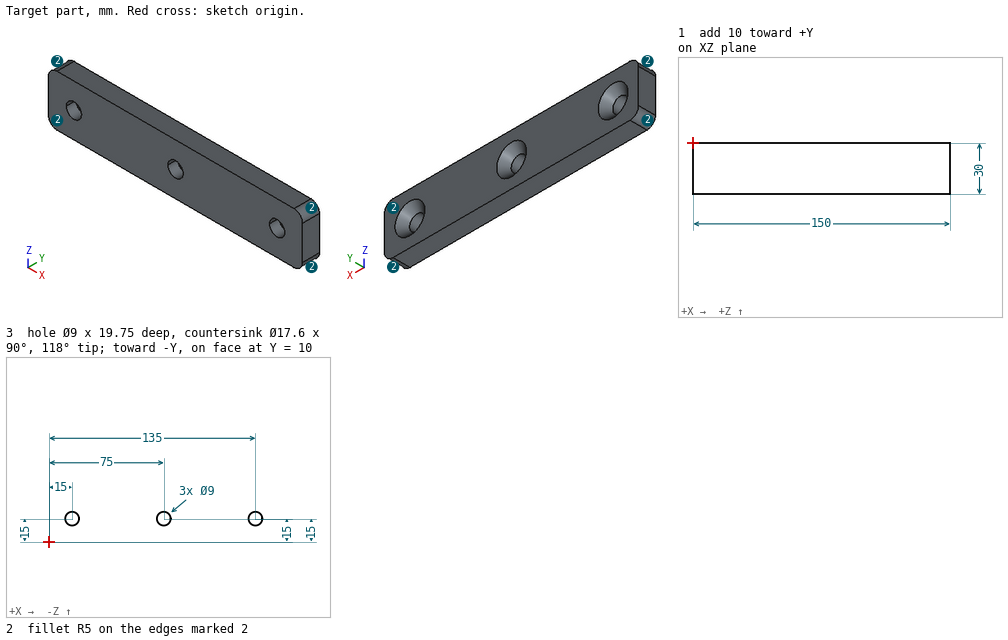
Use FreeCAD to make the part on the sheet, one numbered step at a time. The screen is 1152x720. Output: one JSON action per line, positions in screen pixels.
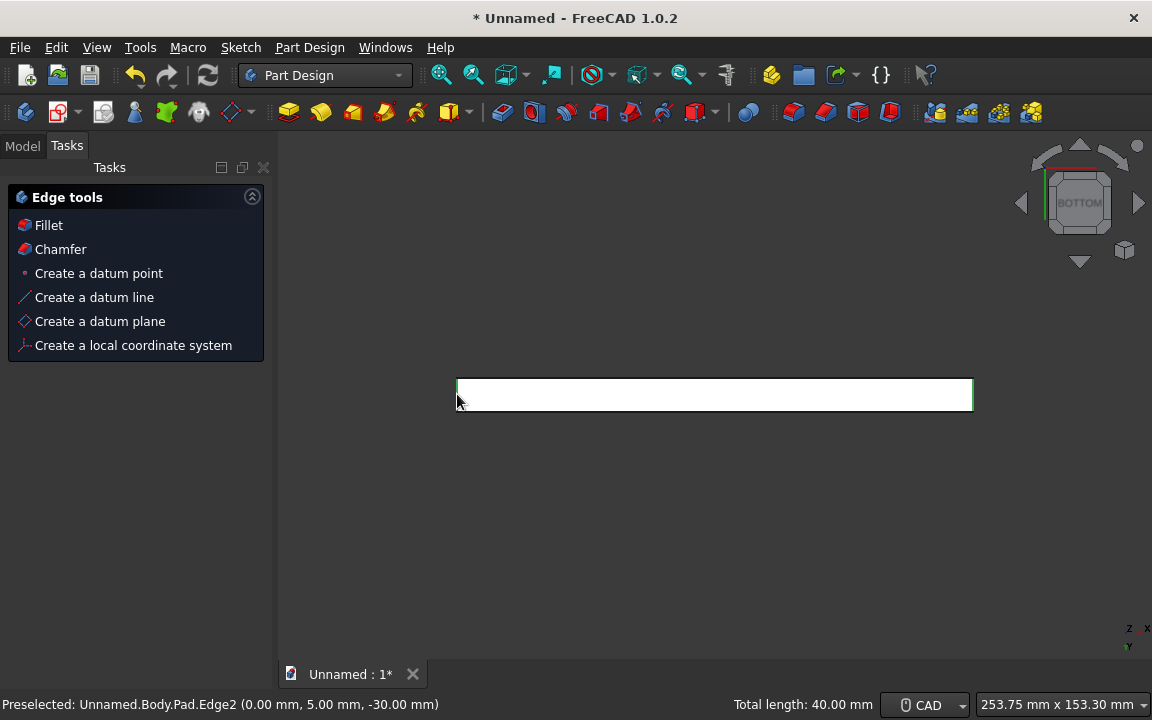
{"action": "left_click", "coordinate": [794, 112]}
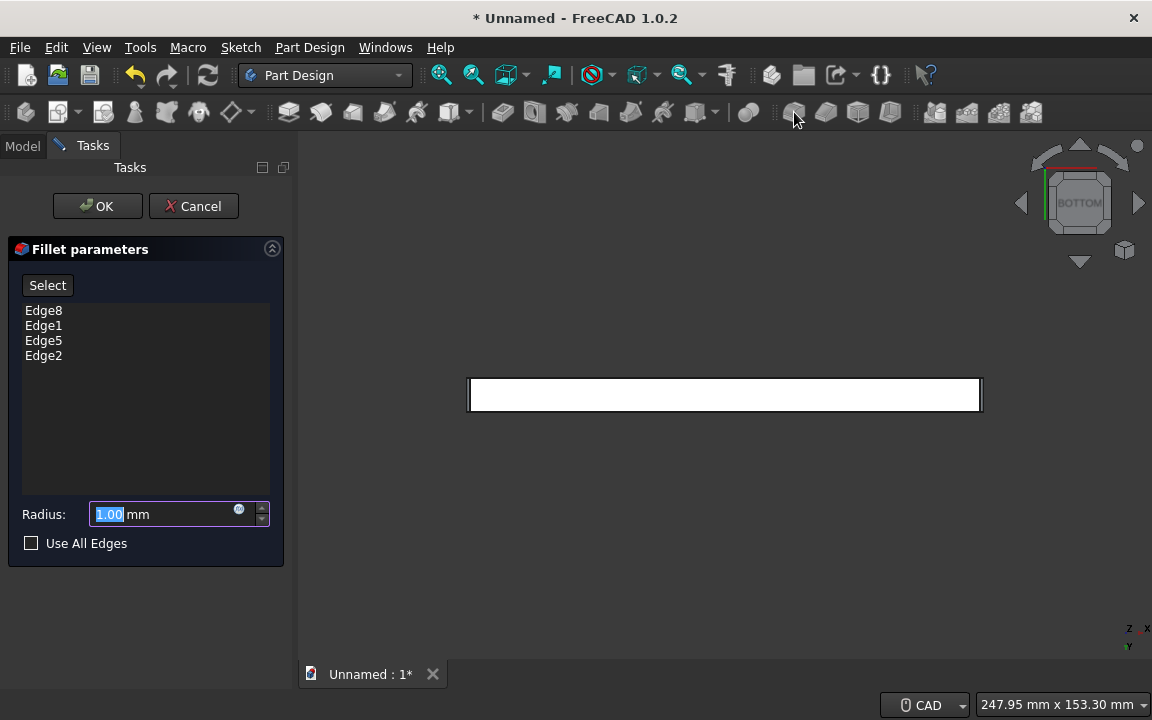
{"action": "type", "text": "5"}
{"action": "key", "text": "Tab"}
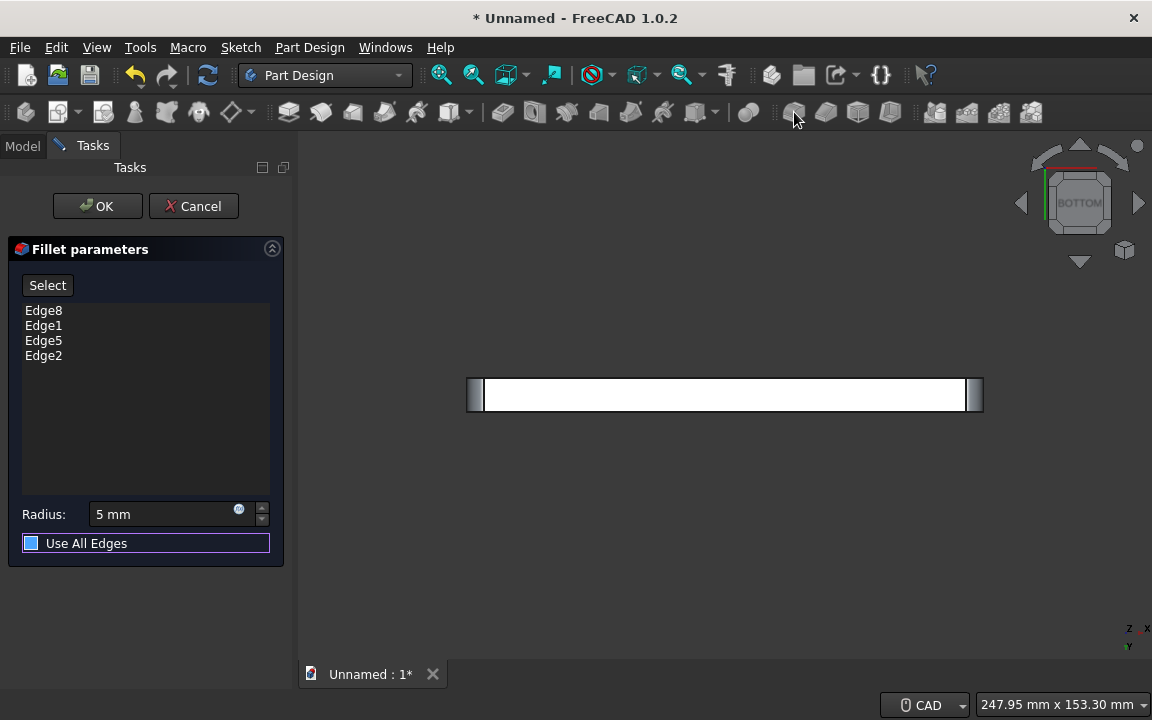
{"action": "left_click", "coordinate": [98, 206]}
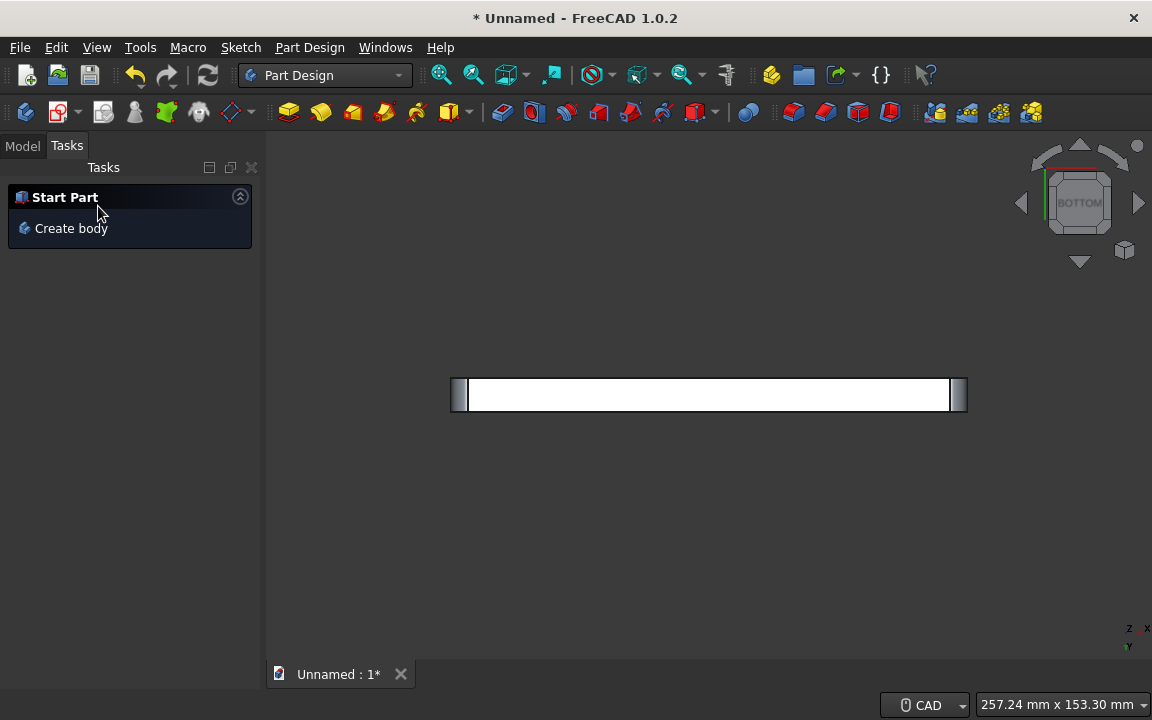
{"action": "key", "text": "4"}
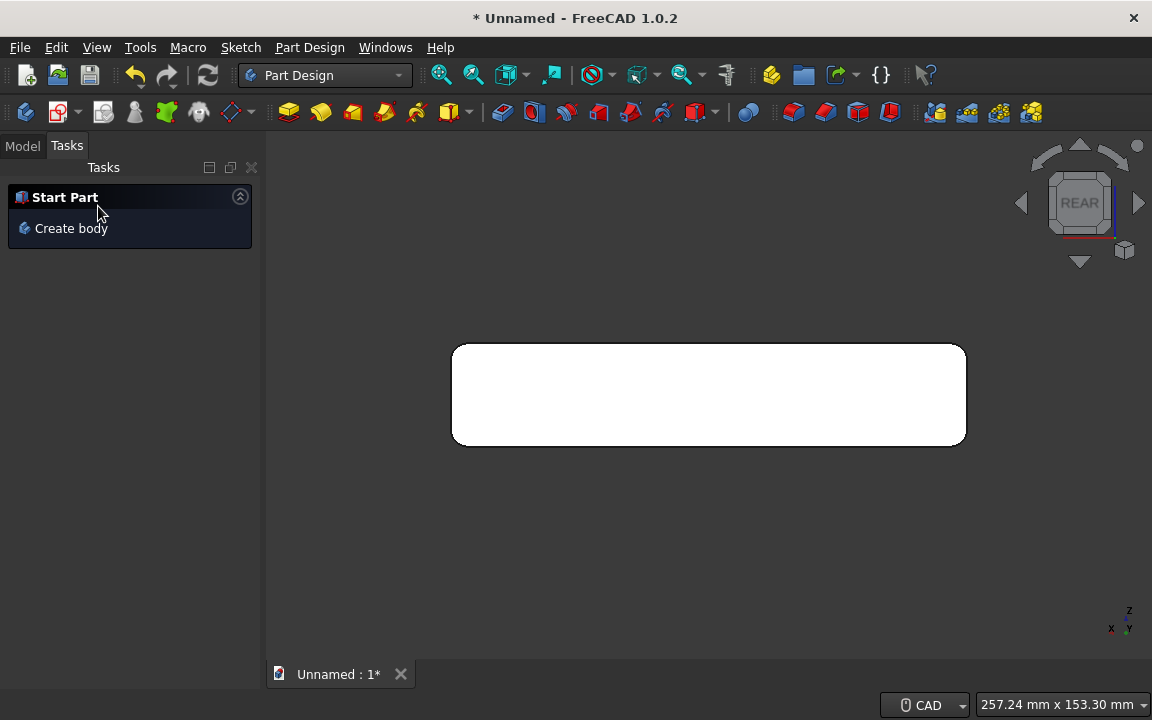
{"action": "left_click", "coordinate": [561, 394]}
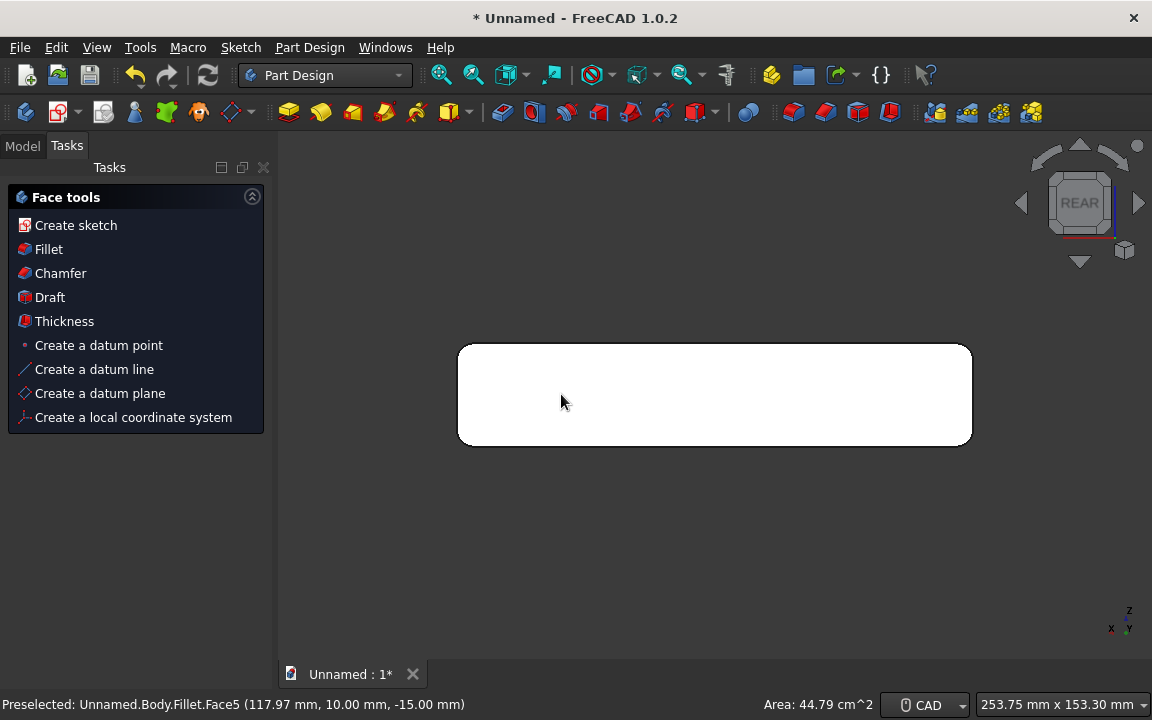
{"action": "left_click", "coordinate": [58, 112]}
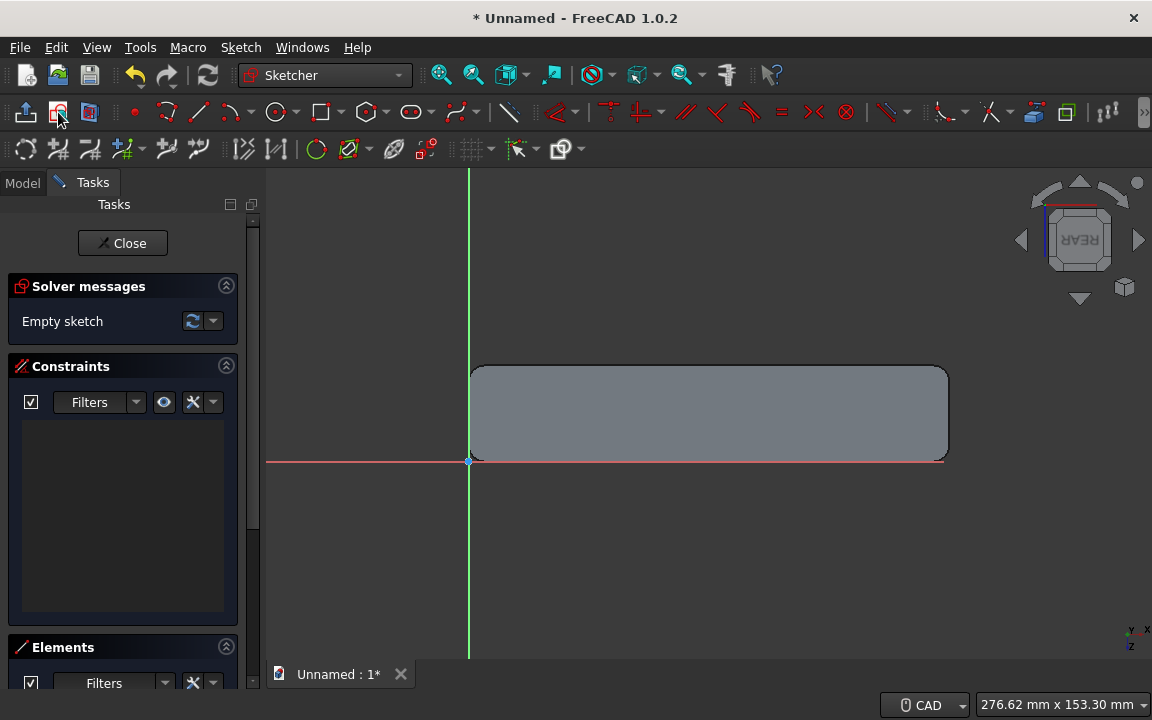
{"action": "left_click", "coordinate": [276, 112]}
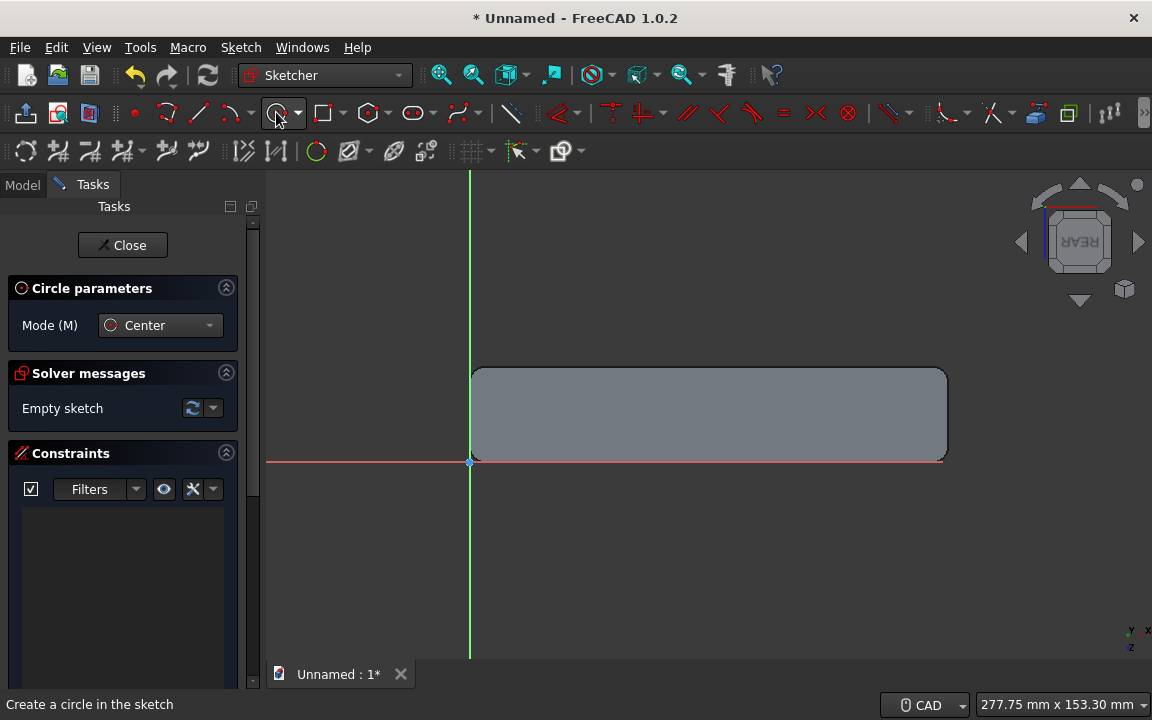
{"action": "scroll", "coordinate": [709, 415], "scroll_direction": "up", "scroll_amount": 3}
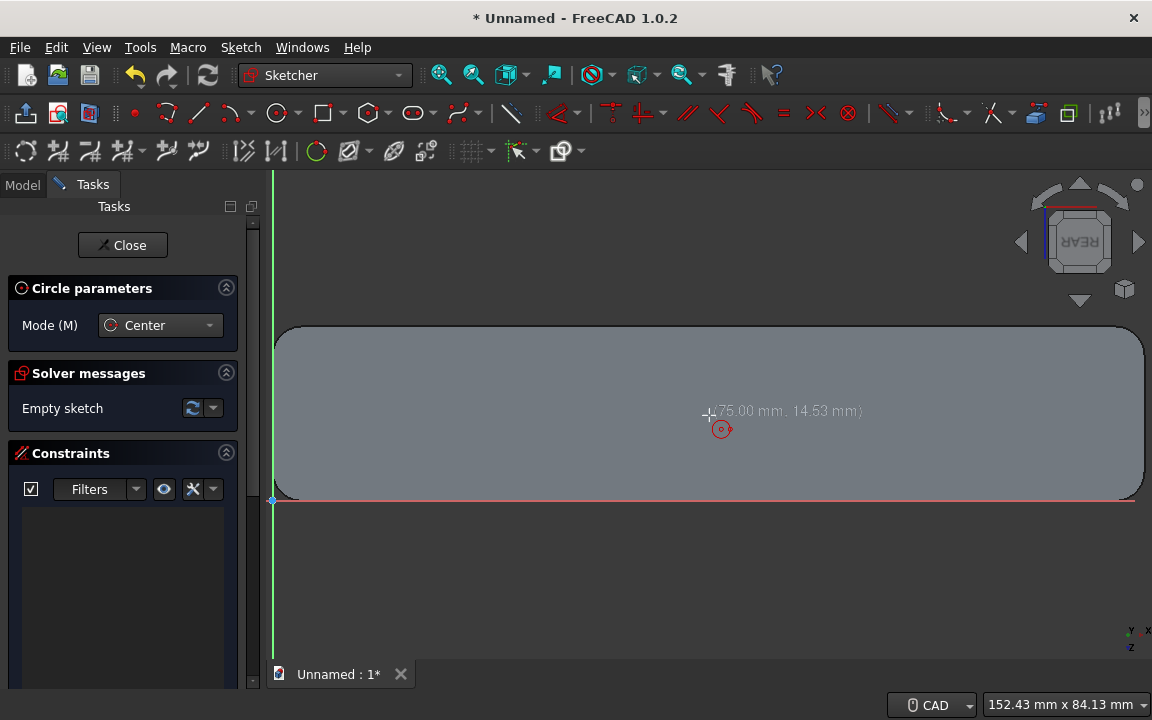
{"action": "left_click", "coordinate": [709, 414]}
{"action": "mouse_move", "coordinate": [727, 395]}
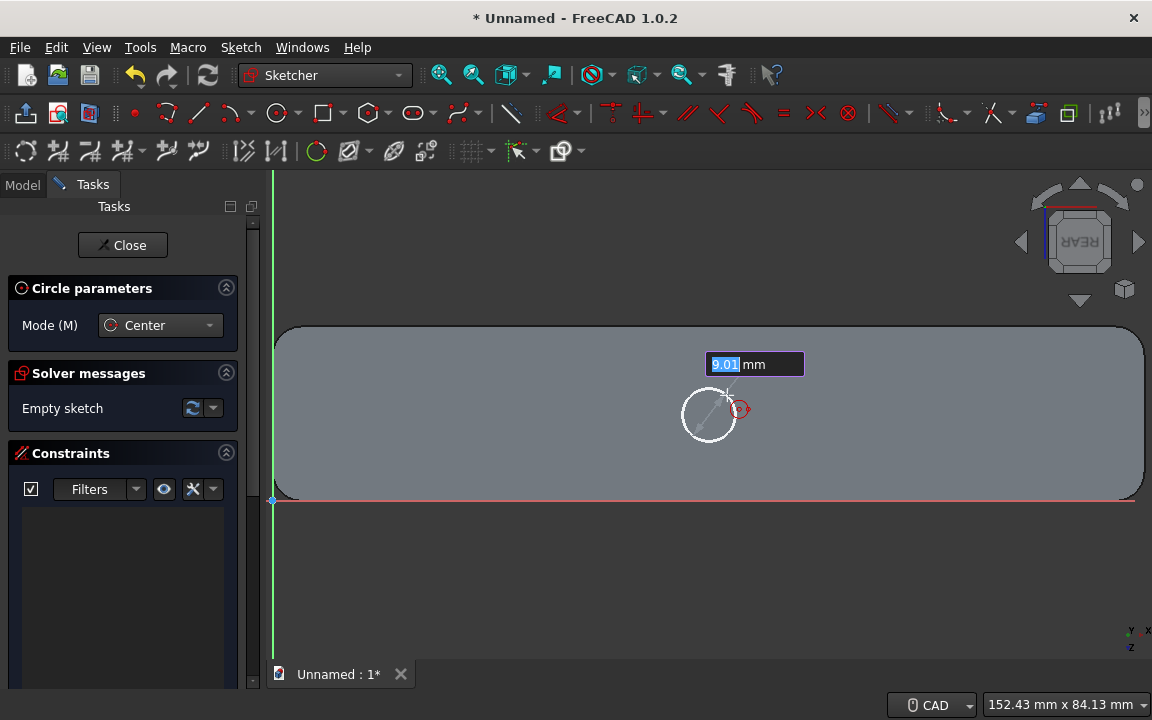
{"action": "type", "text": "9"}
{"action": "key", "text": "Return"}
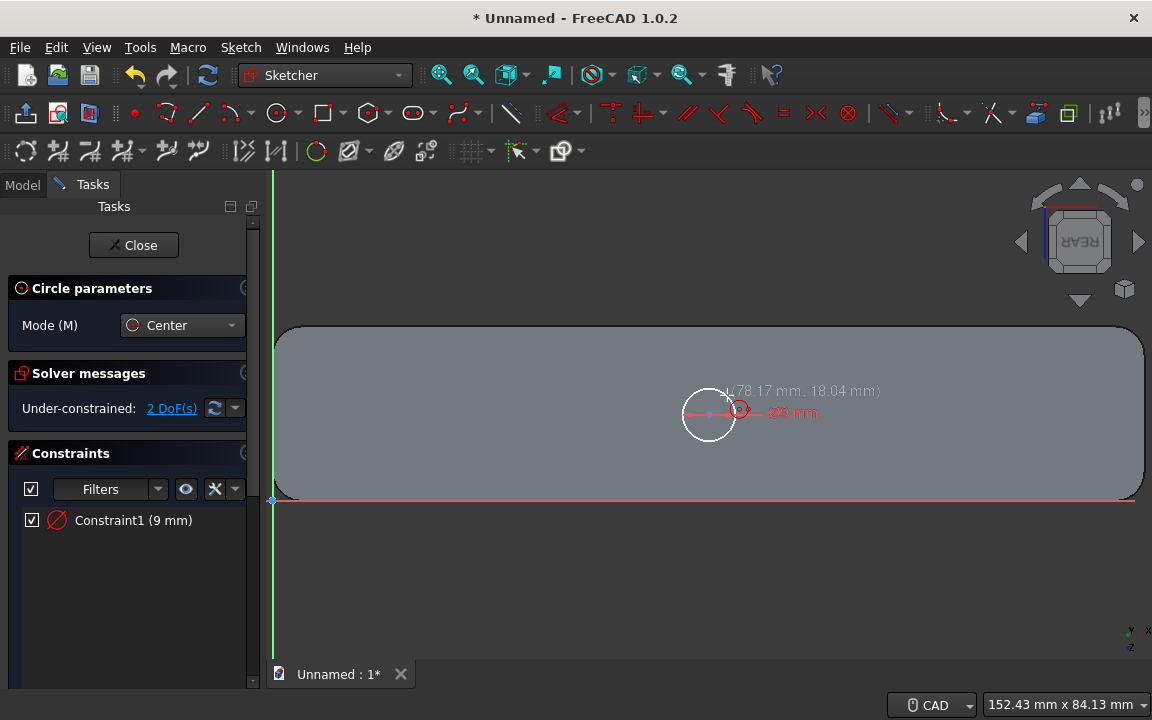
{"action": "left_click", "coordinate": [360, 414]}
{"action": "mouse_move", "coordinate": [378, 395]}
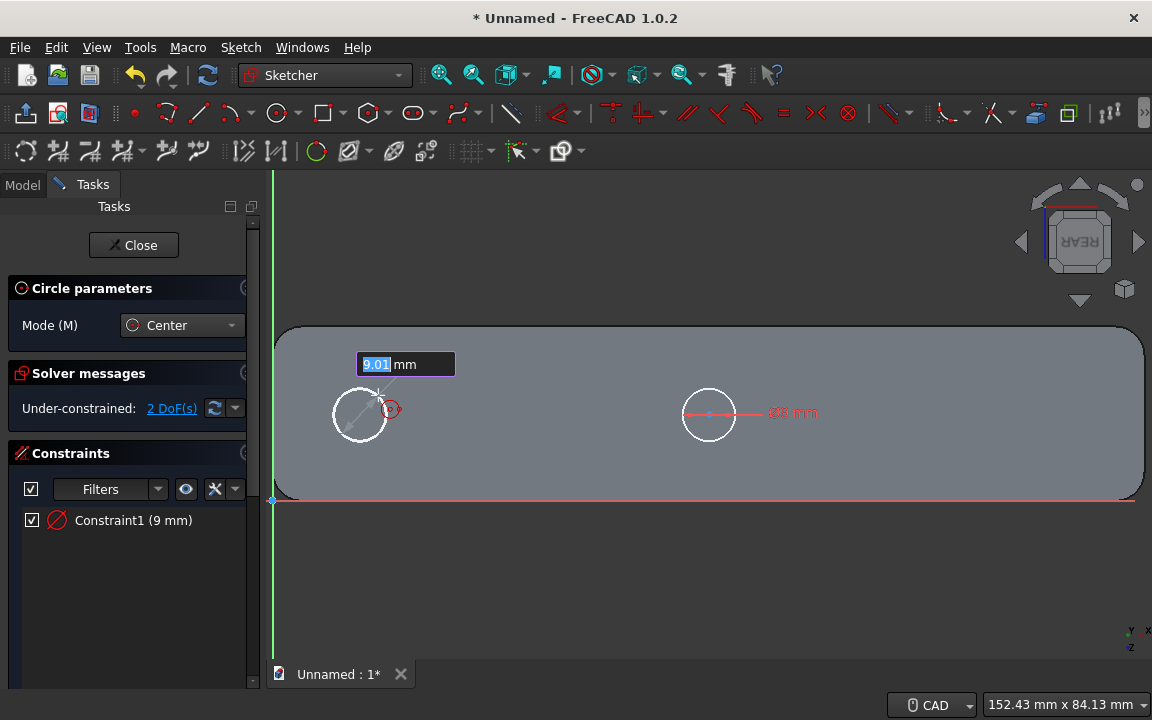
{"action": "type", "text": "9"}
{"action": "key", "text": "Return"}